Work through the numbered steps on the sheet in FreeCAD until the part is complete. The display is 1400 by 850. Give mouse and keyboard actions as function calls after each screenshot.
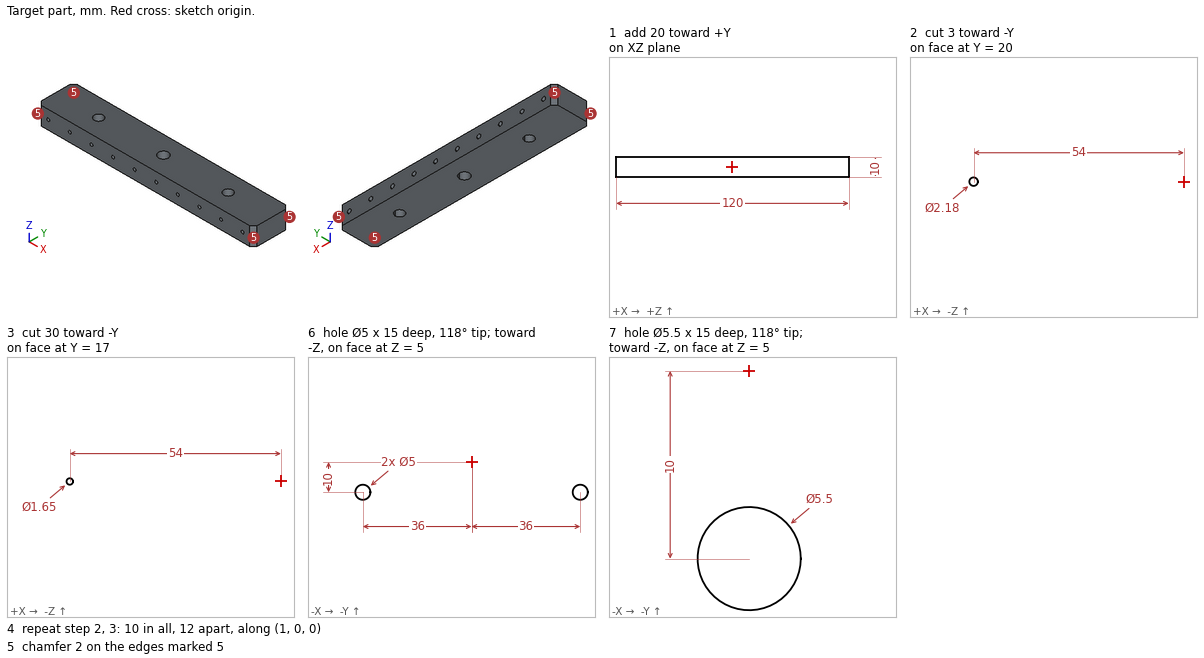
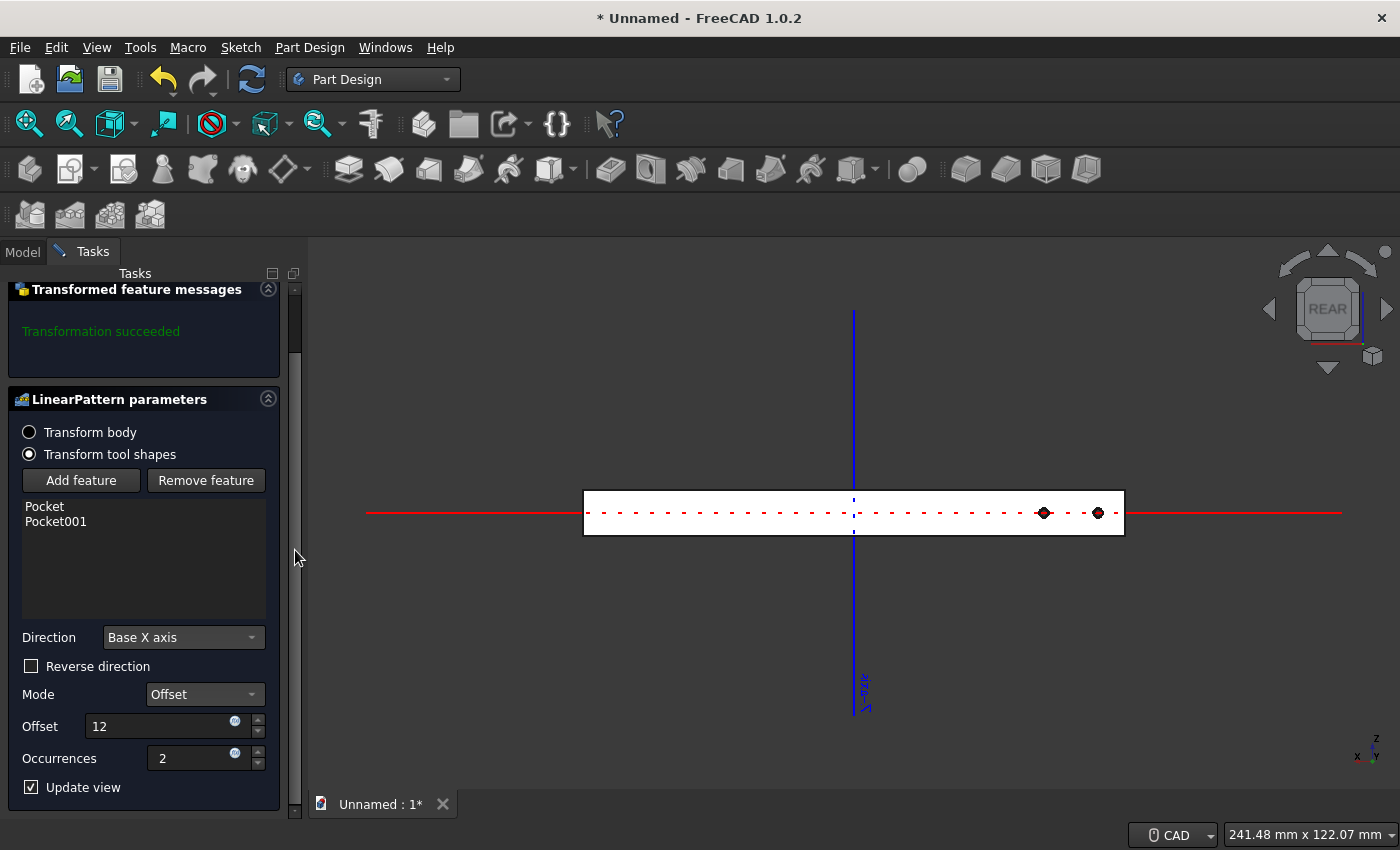
triple_click(198, 758)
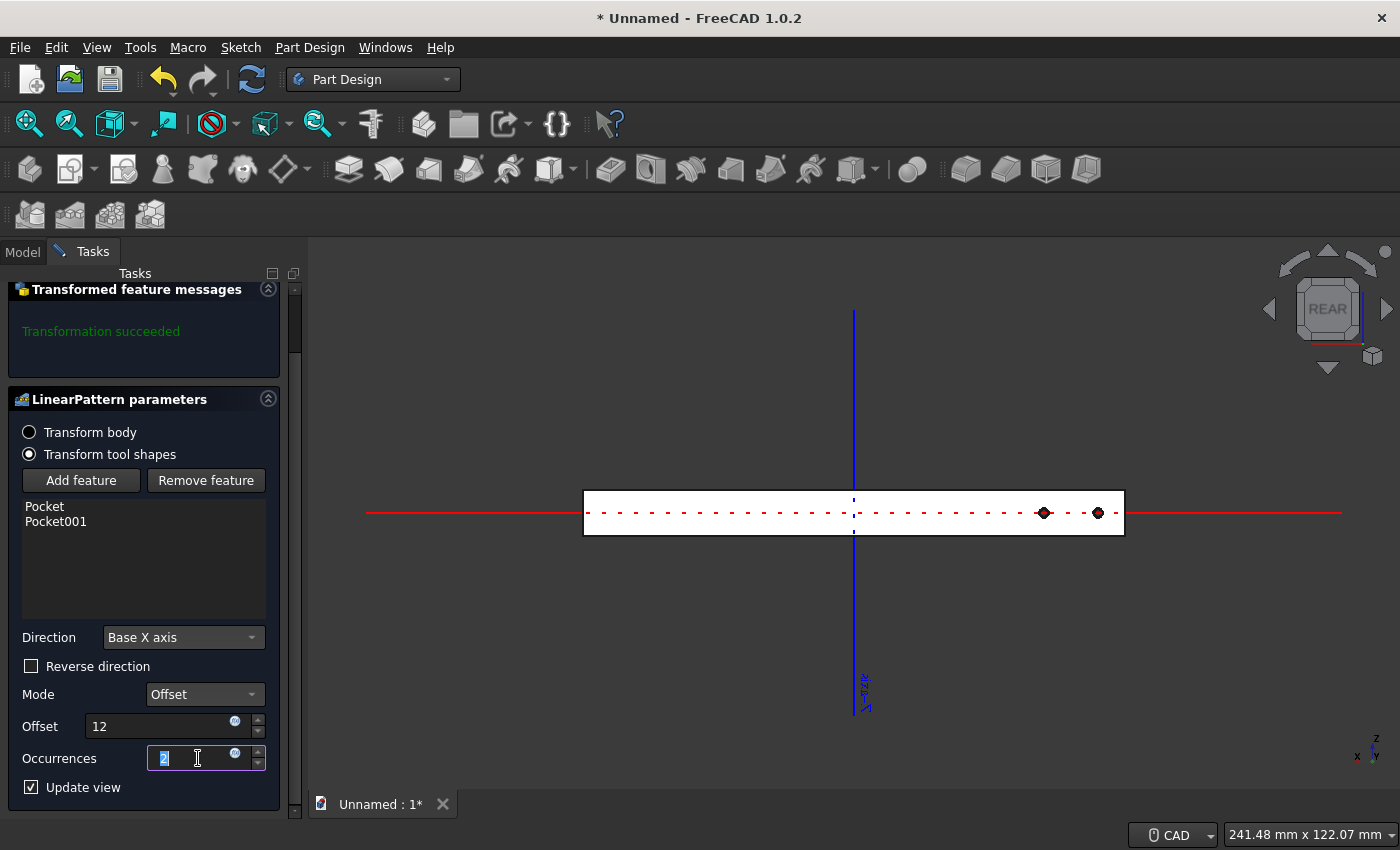
text(10)
key(Tab)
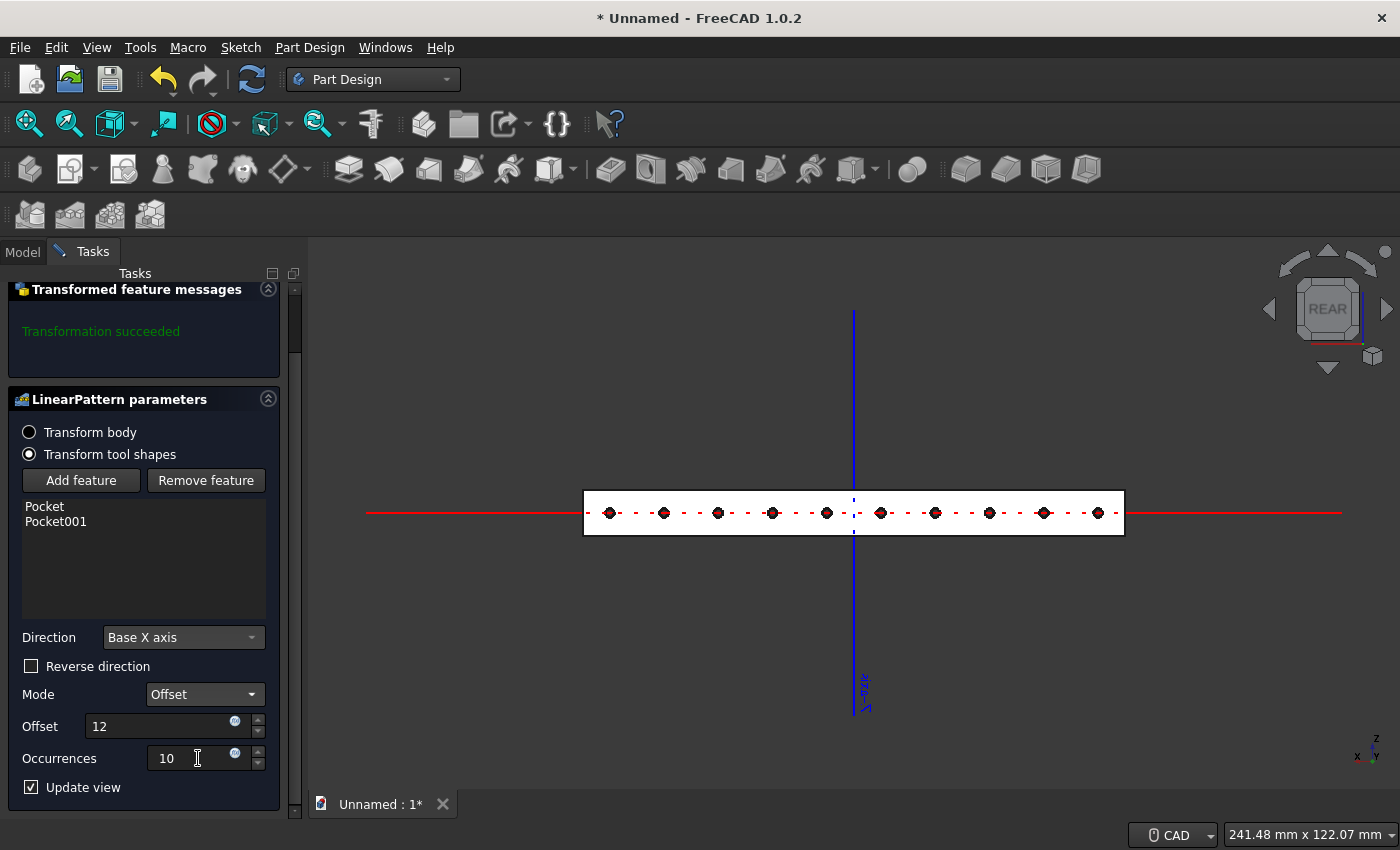
scroll(295, 550, up, 2)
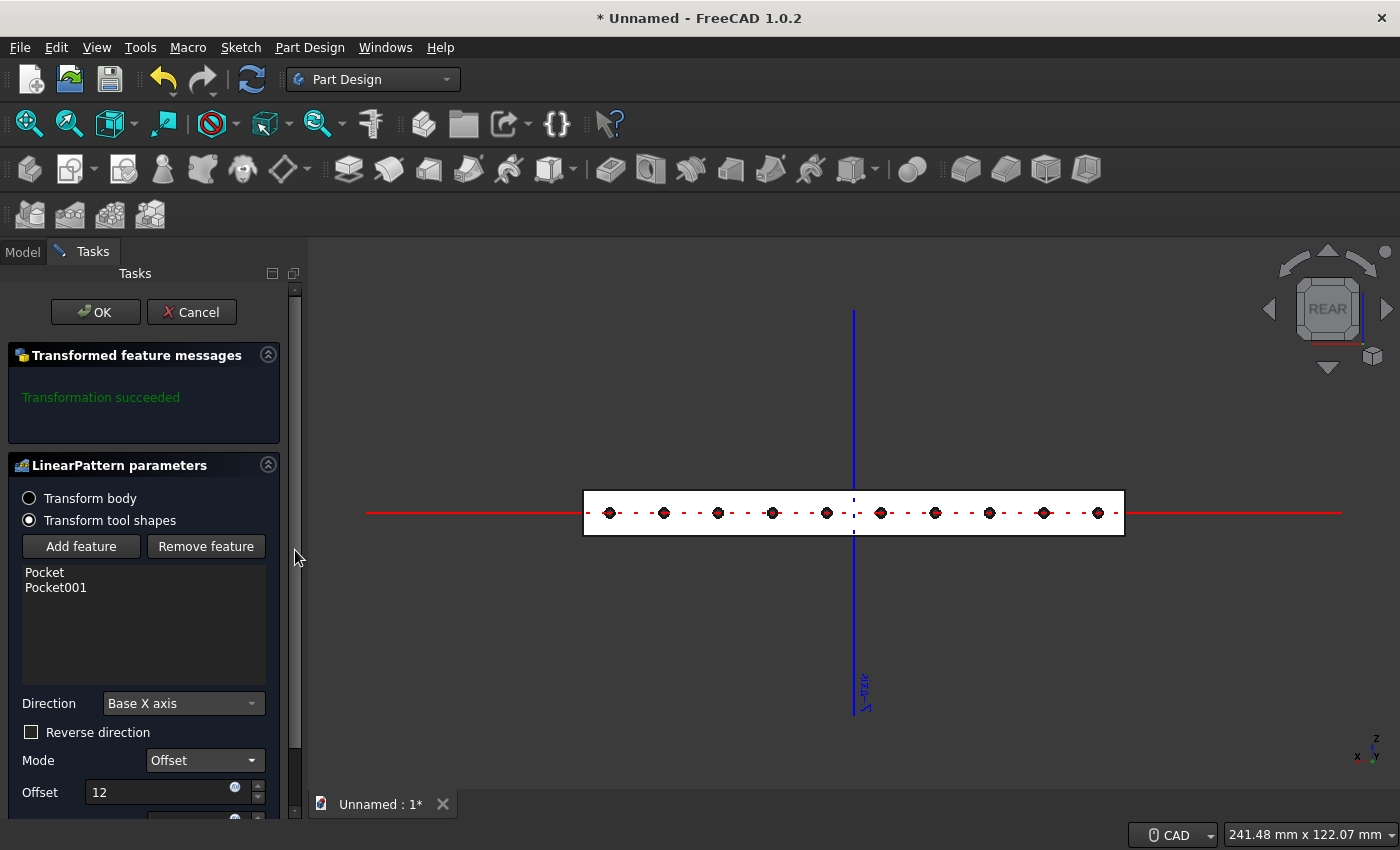
click(96, 312)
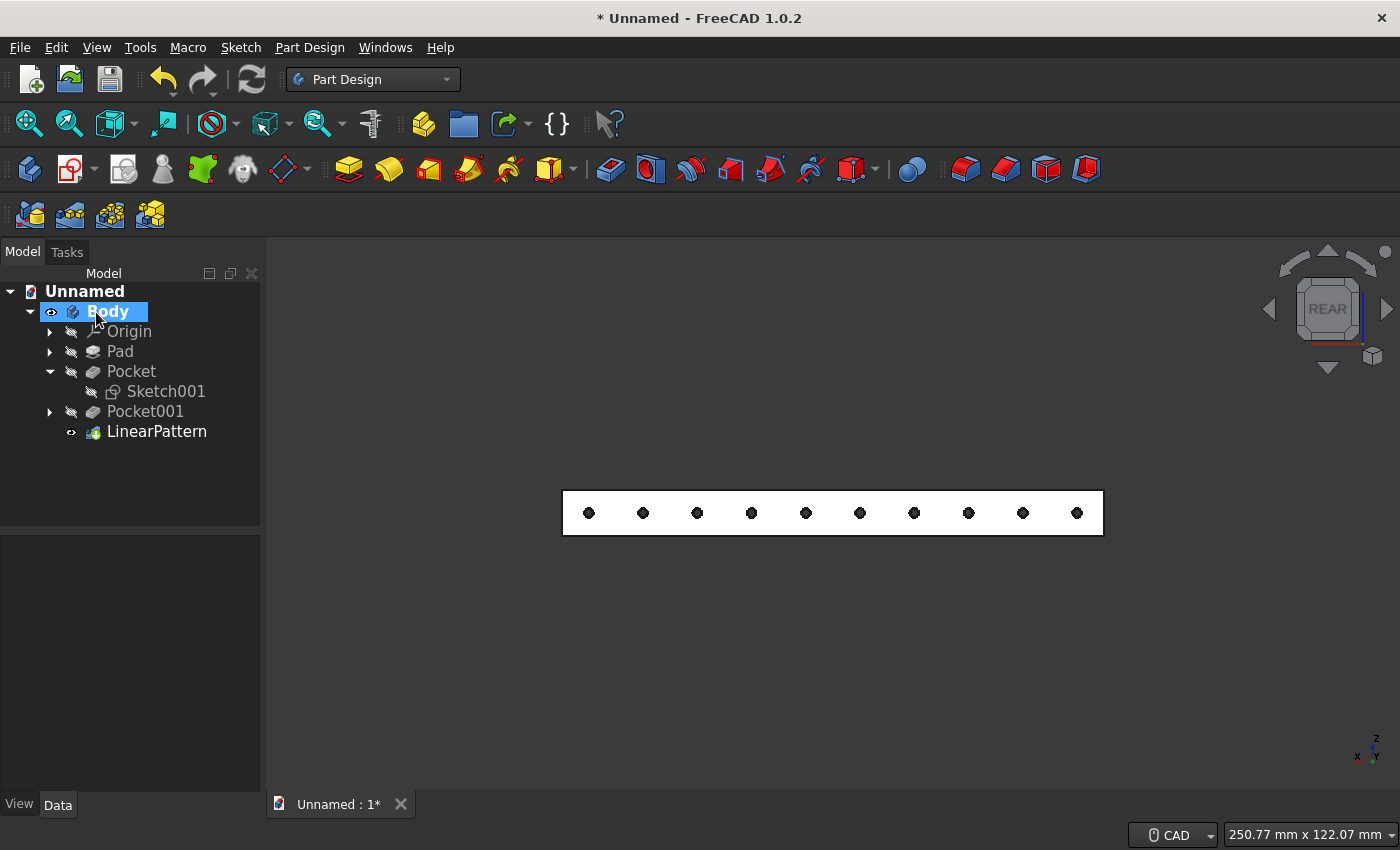
click(1104, 512)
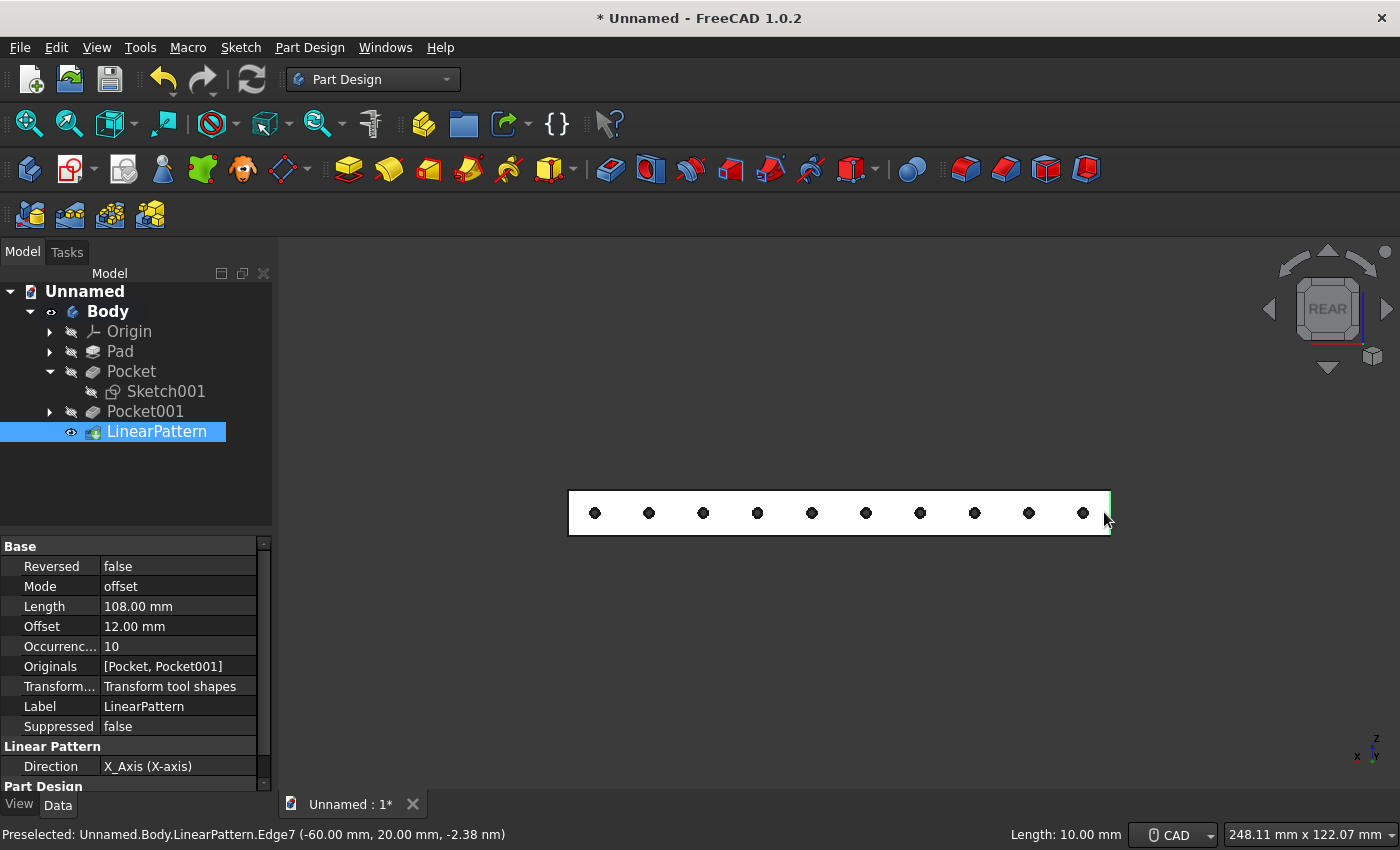
key(0)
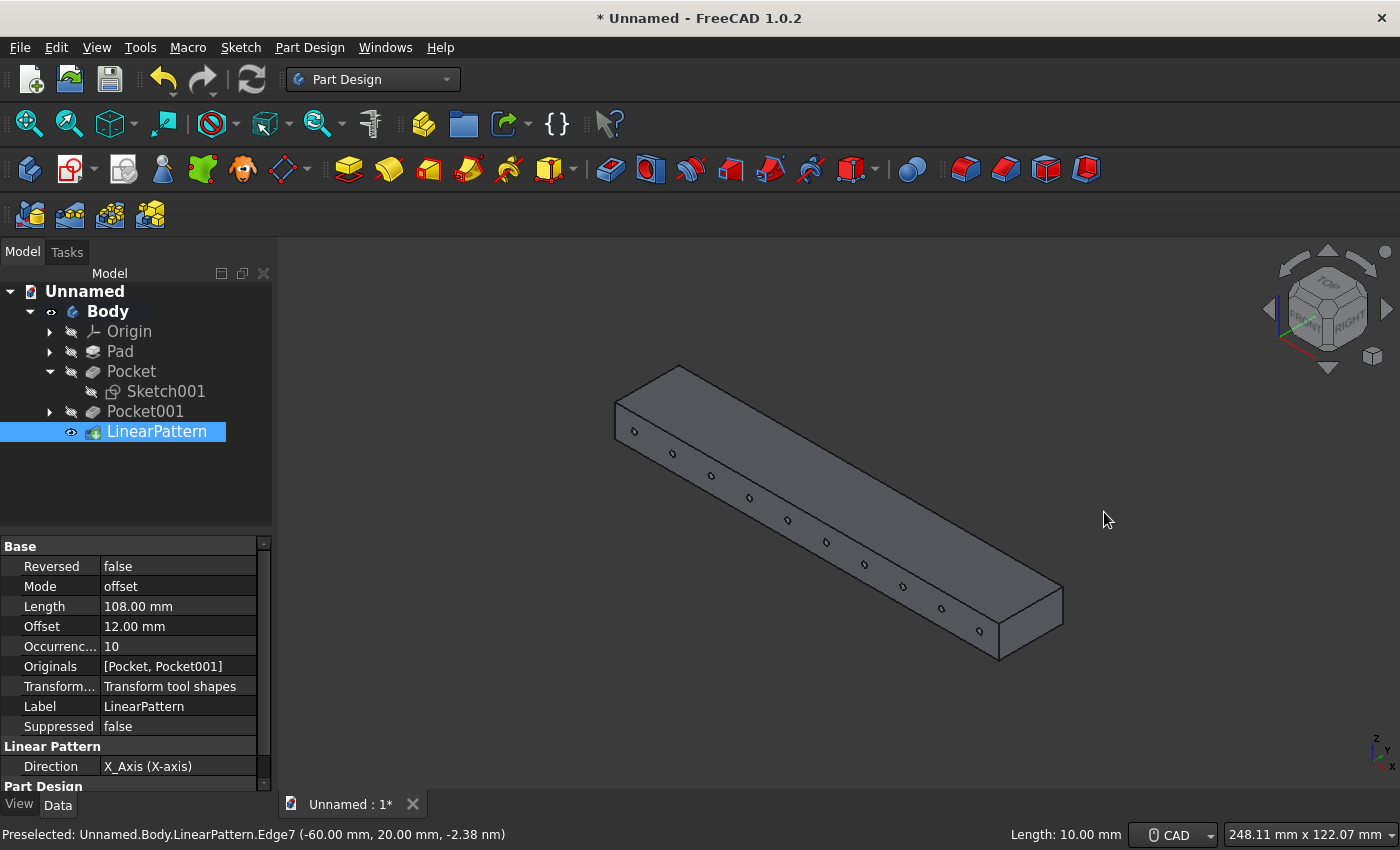
click(999, 641, ctrl)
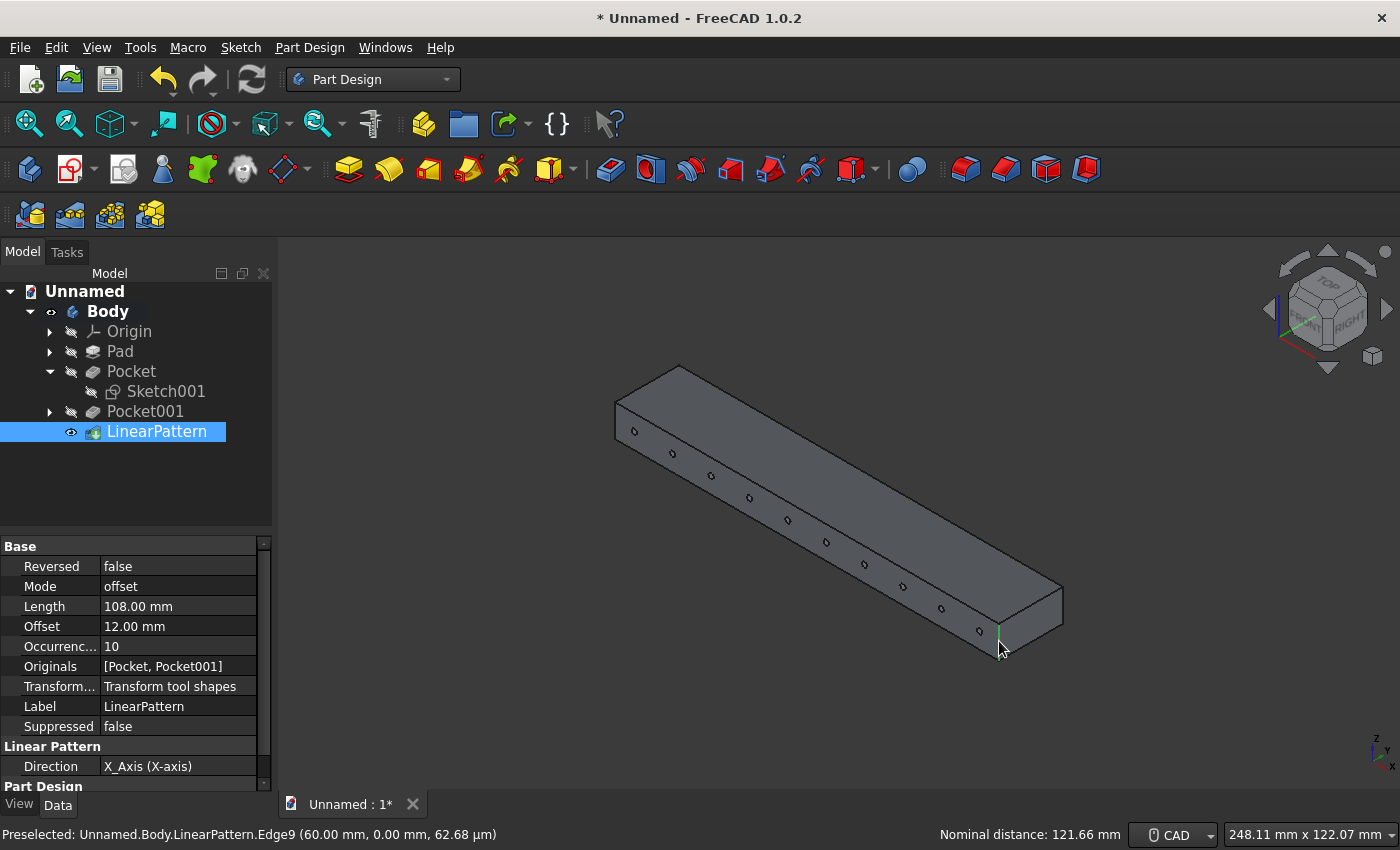
key(2)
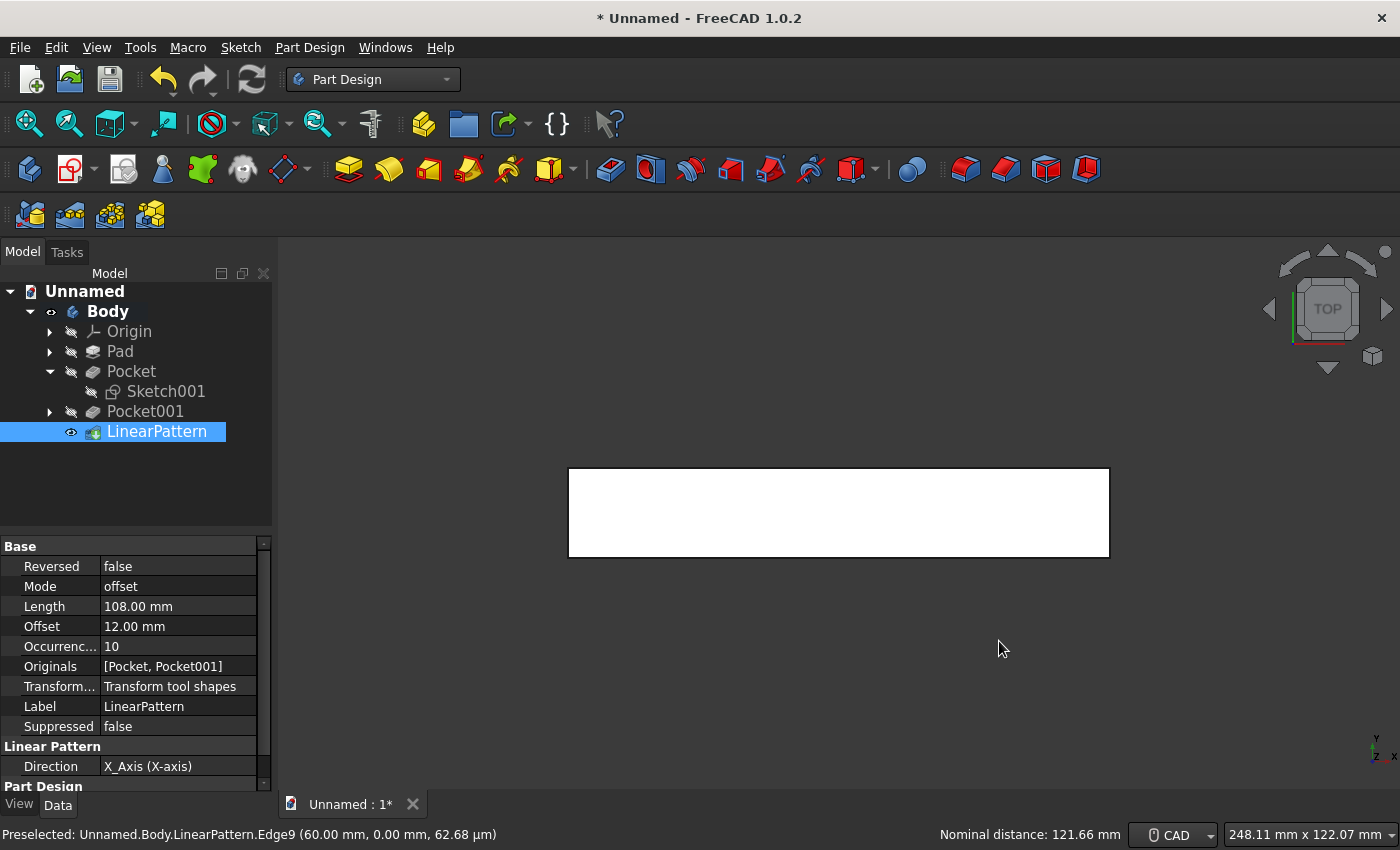
key(1)